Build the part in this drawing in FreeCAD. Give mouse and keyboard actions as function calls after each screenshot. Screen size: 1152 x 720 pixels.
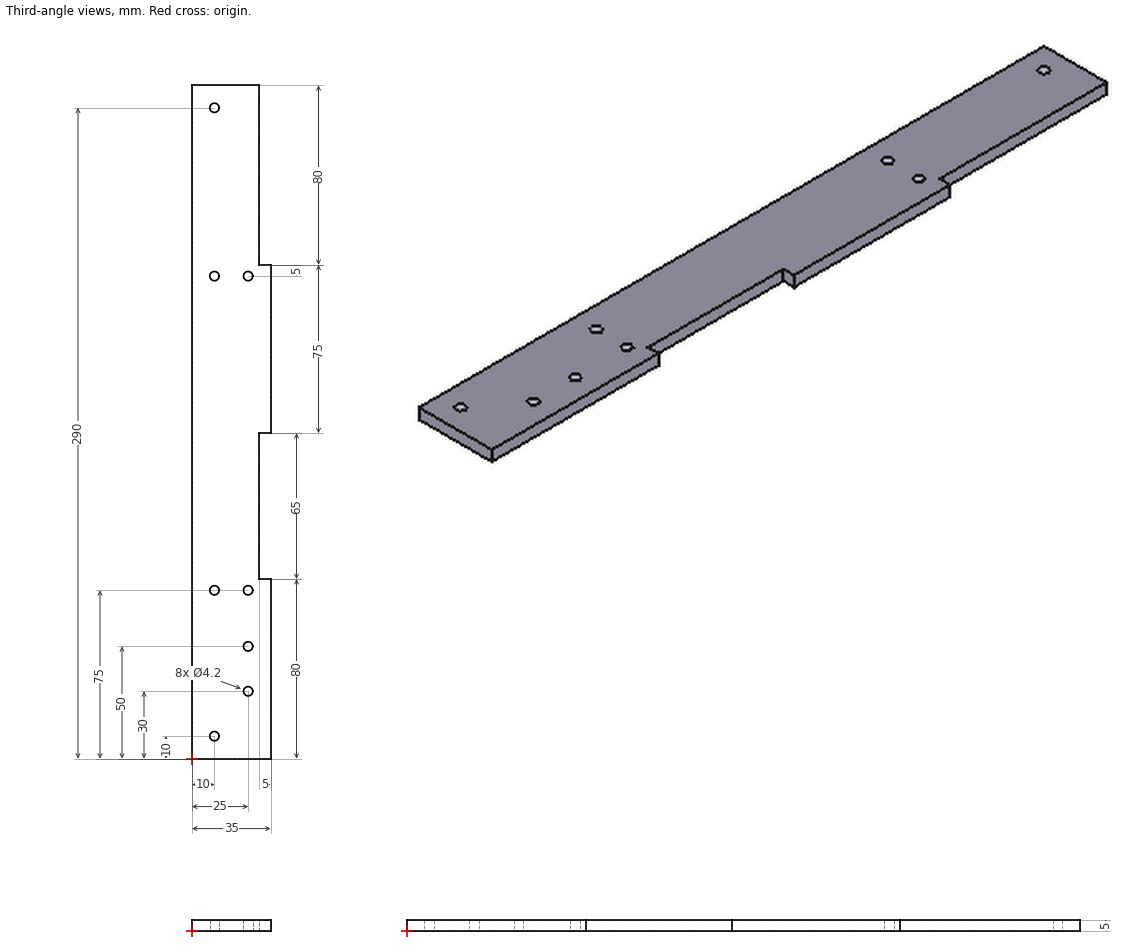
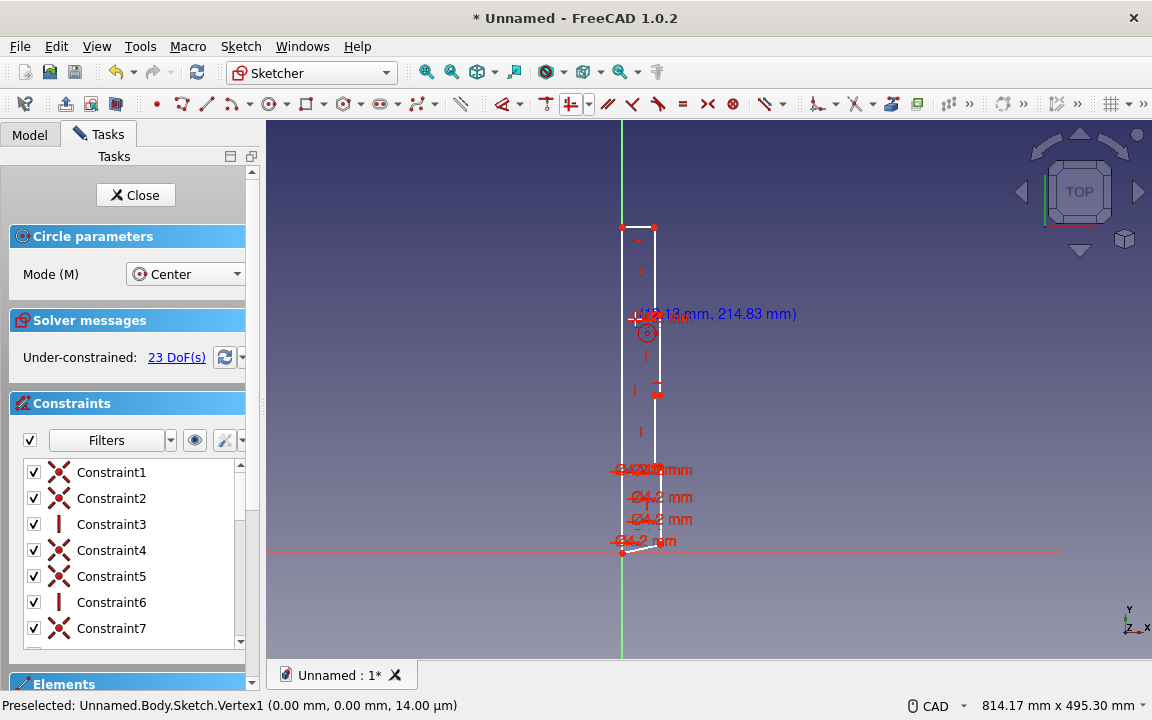
scroll(633, 319, up, 2)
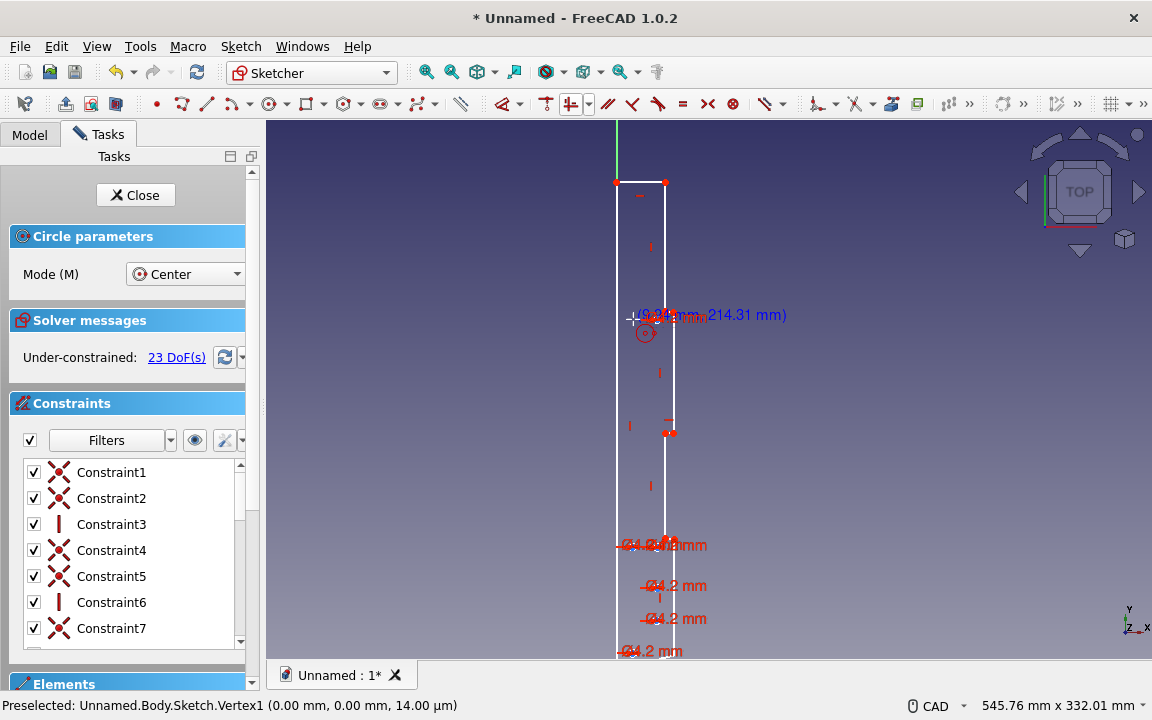
click(633, 319)
move(635, 317)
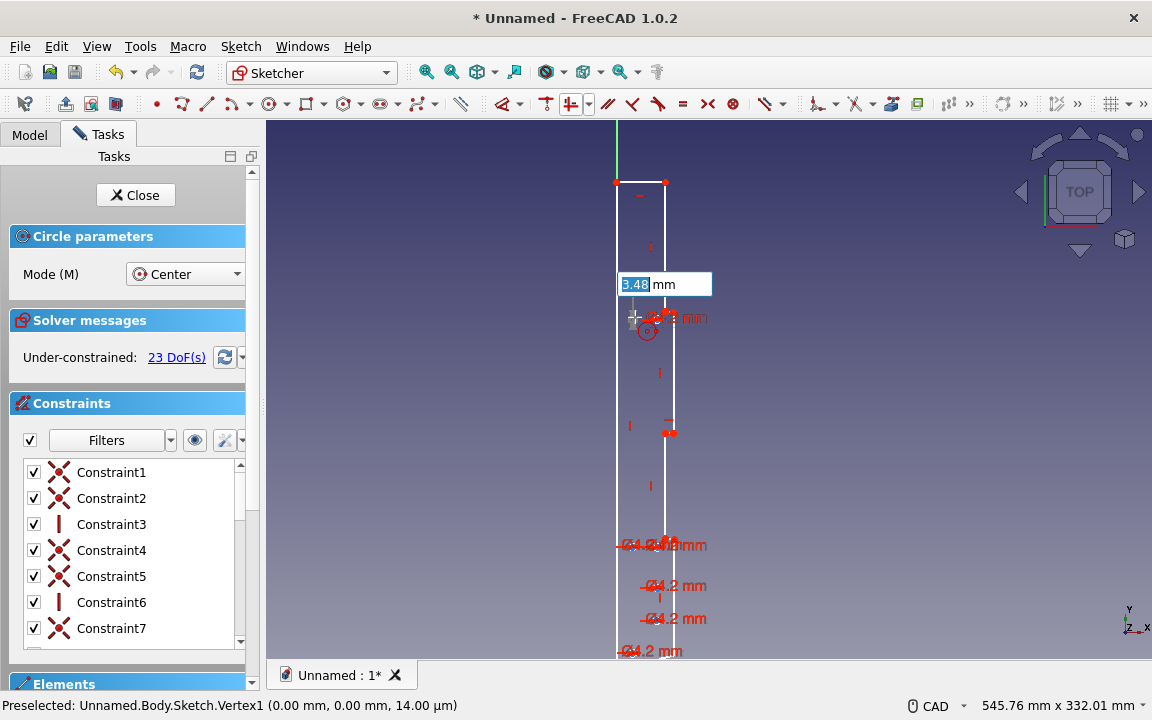
text(4.2)
key(Return)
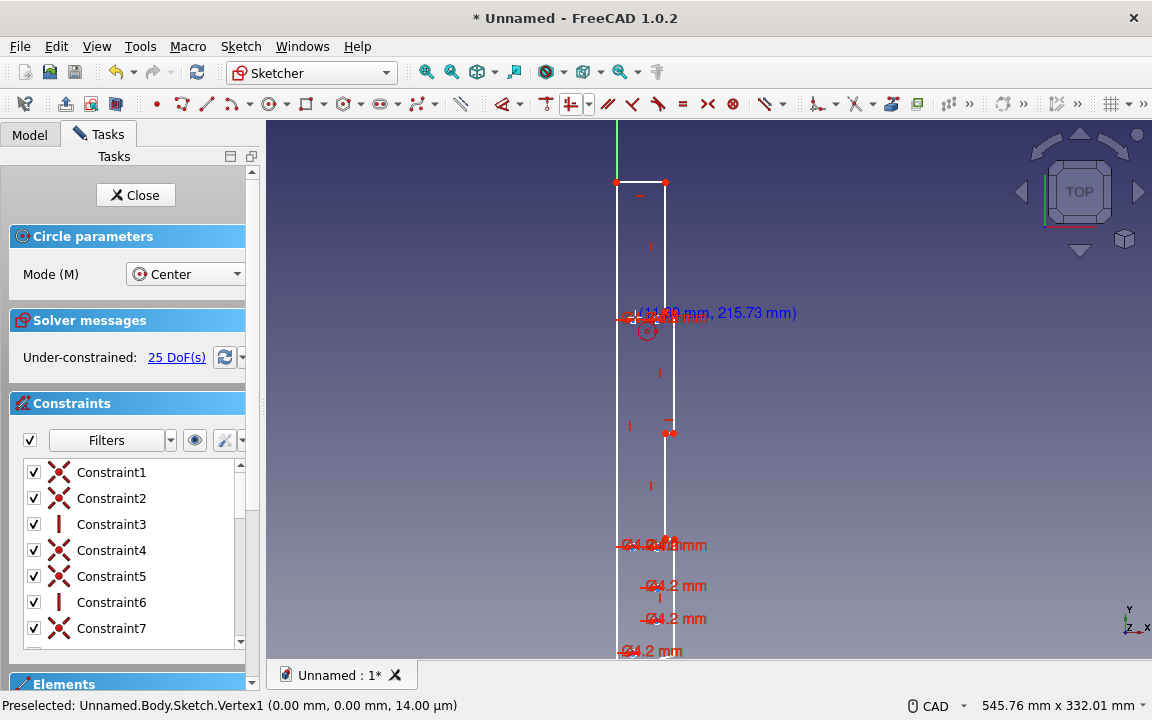
scroll(633, 197, up, 10)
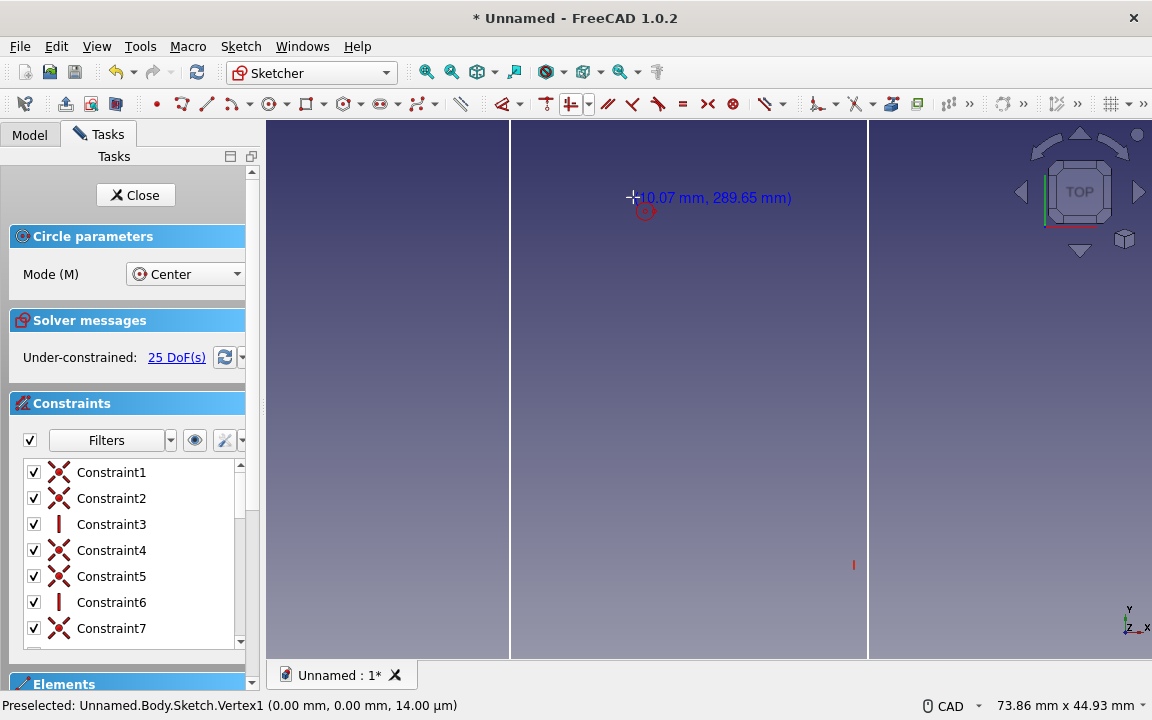
scroll(633, 241, down, 12)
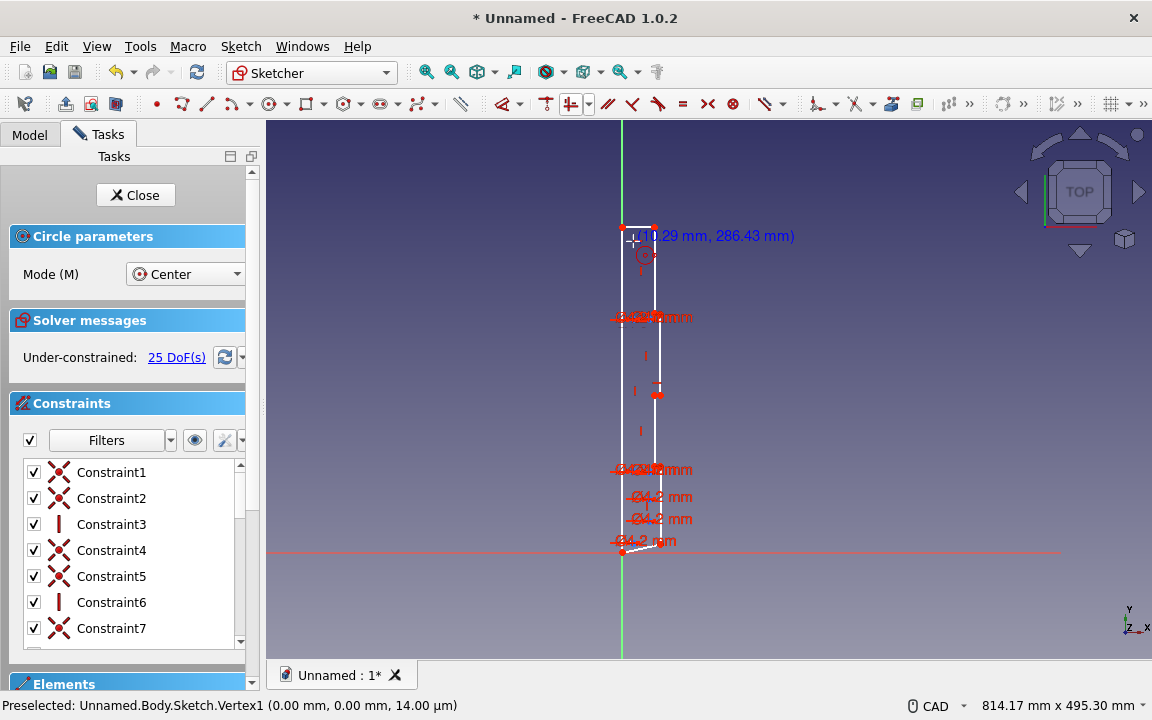
scroll(633, 237, up, 2)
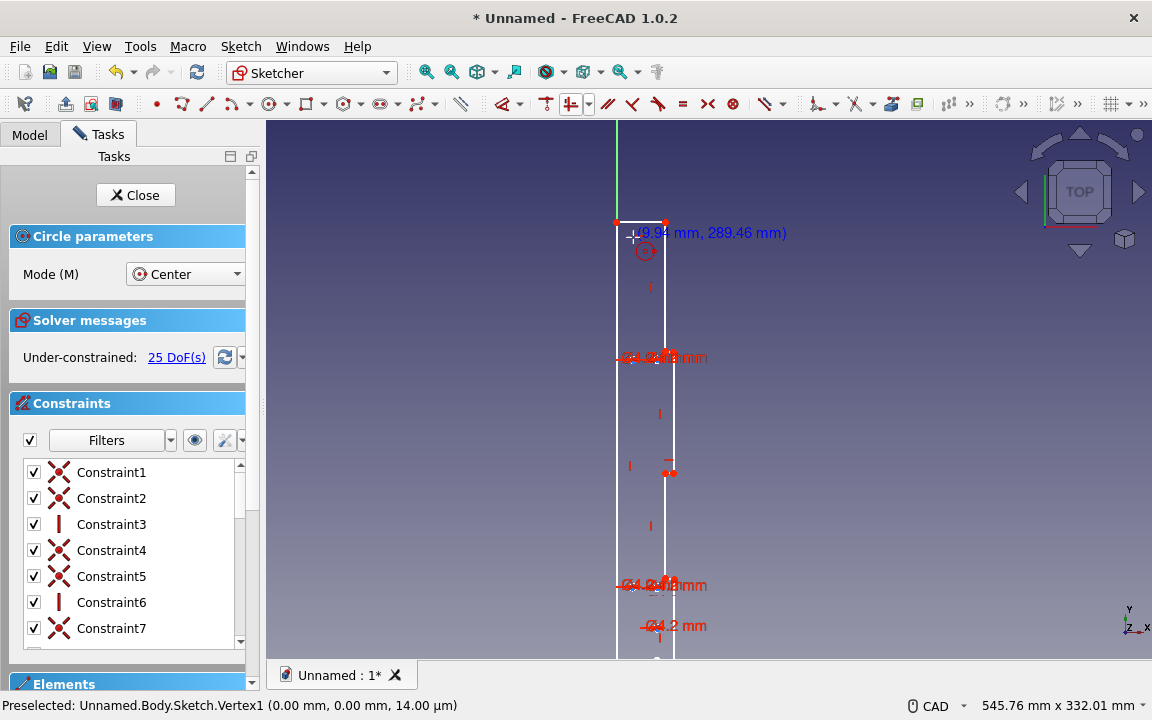
click(633, 238)
move(635, 240)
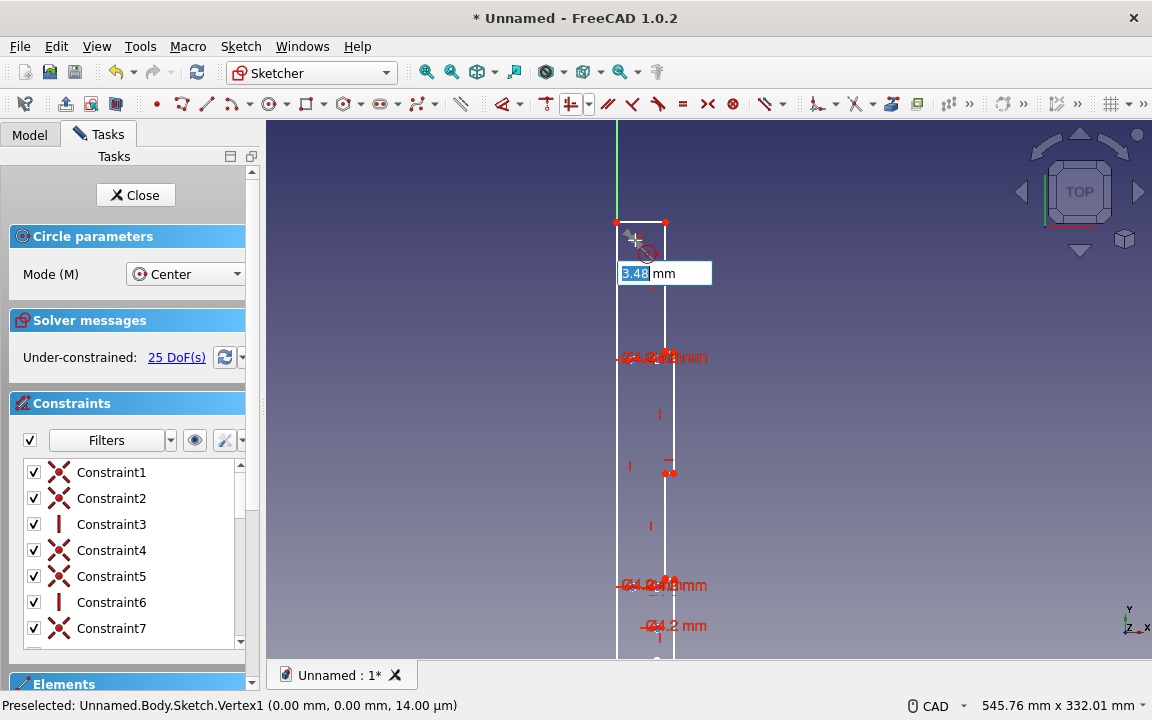
text(4.2)
key(Return)
key(Escape)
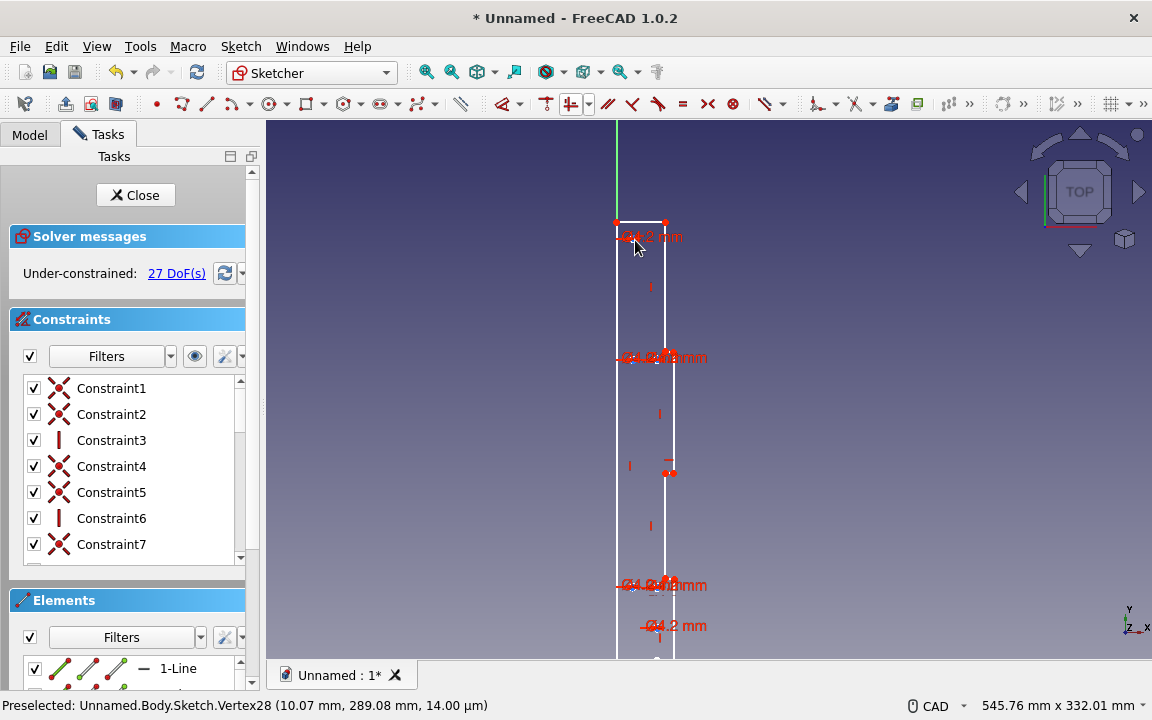
scroll(631, 236, down, 2)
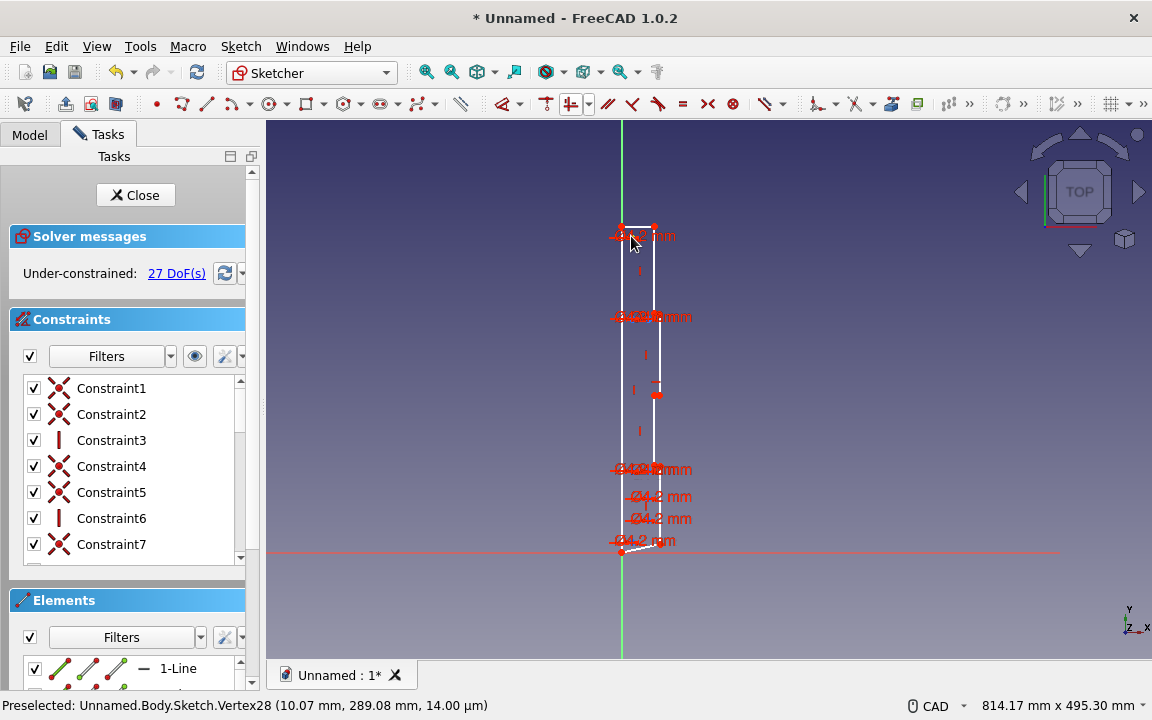
scroll(629, 551, up, 4)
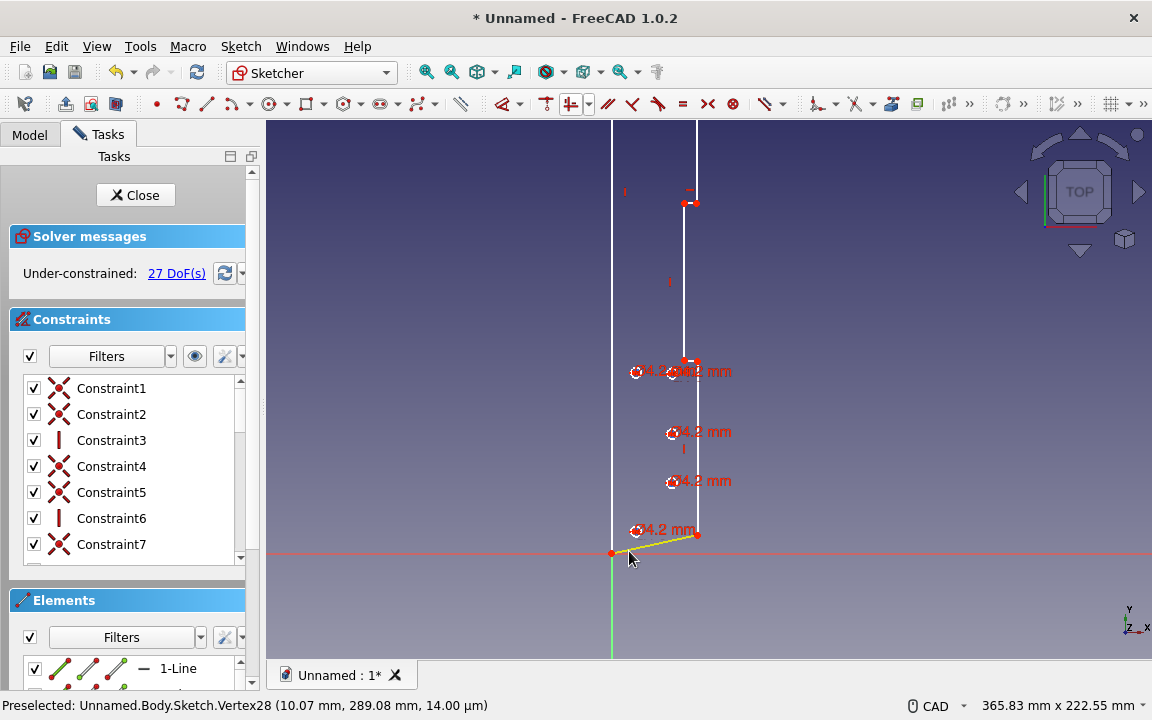
click(629, 550)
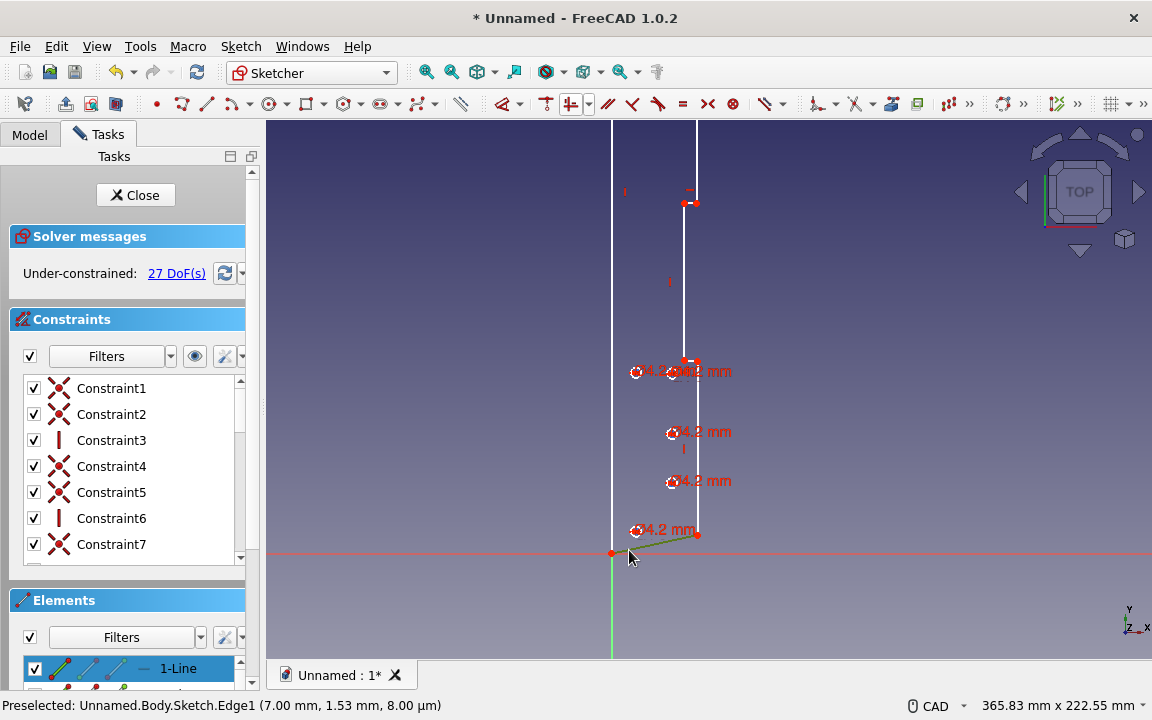
click(588, 104)